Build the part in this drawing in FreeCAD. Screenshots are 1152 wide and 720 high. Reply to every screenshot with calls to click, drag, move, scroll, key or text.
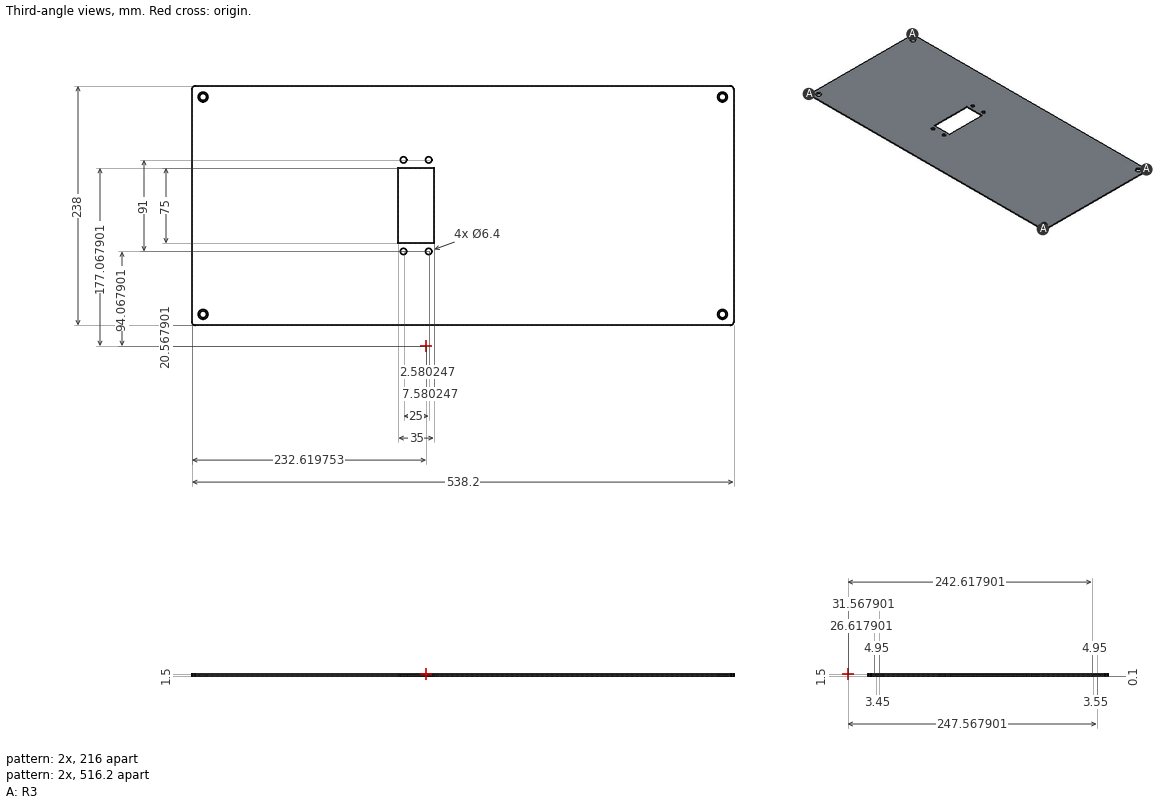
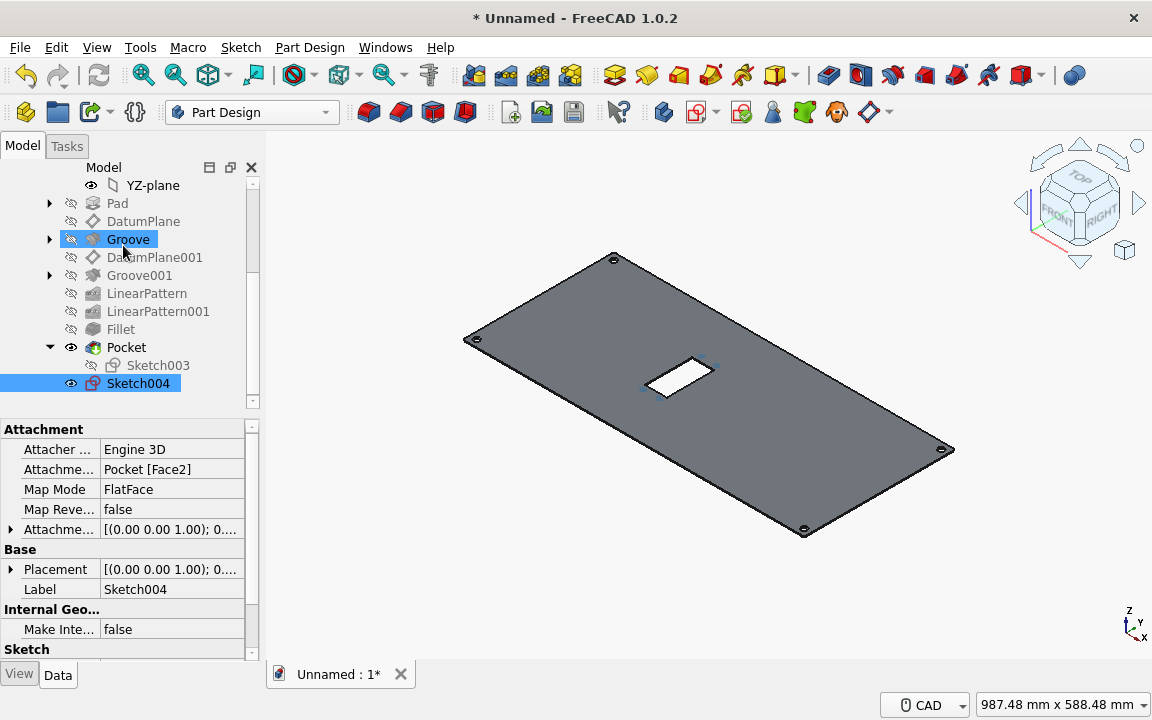
click(830, 76)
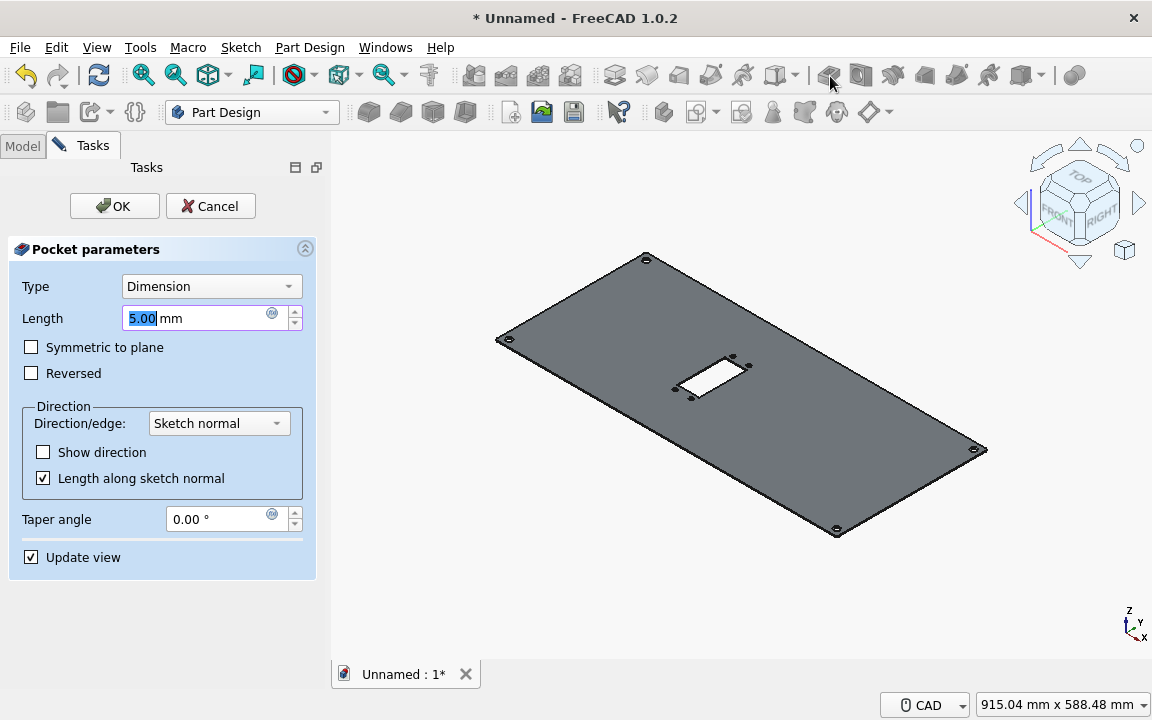
text(1.5)
key(Tab)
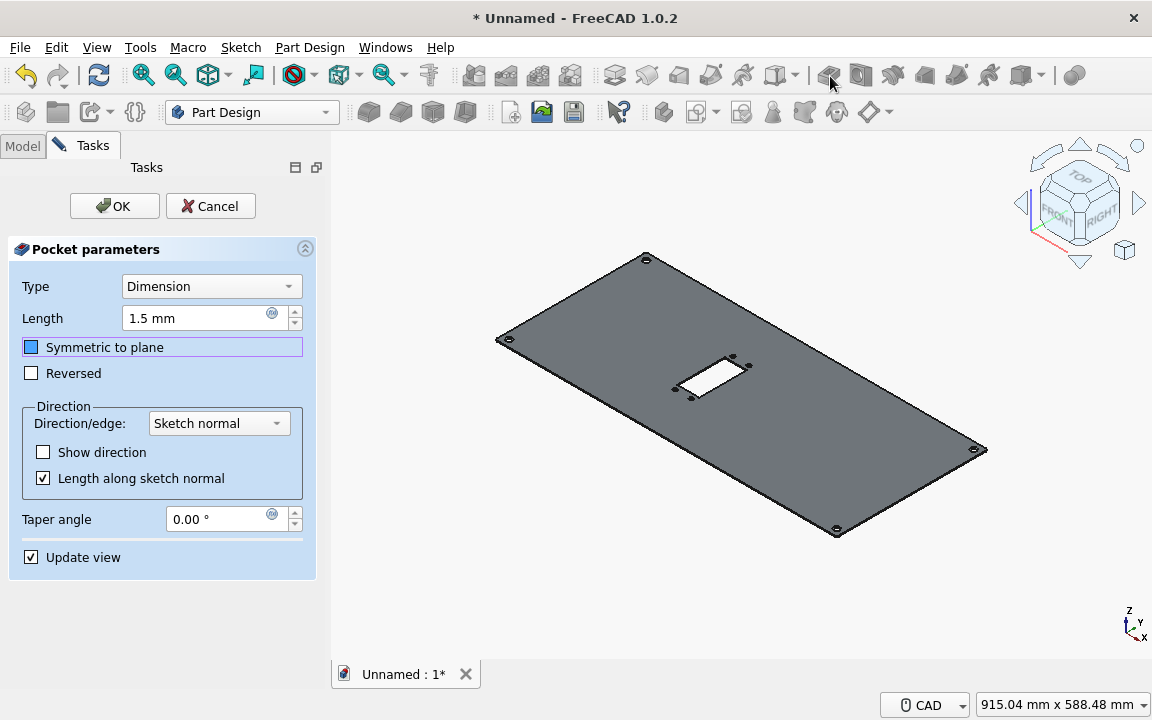
click(115, 206)